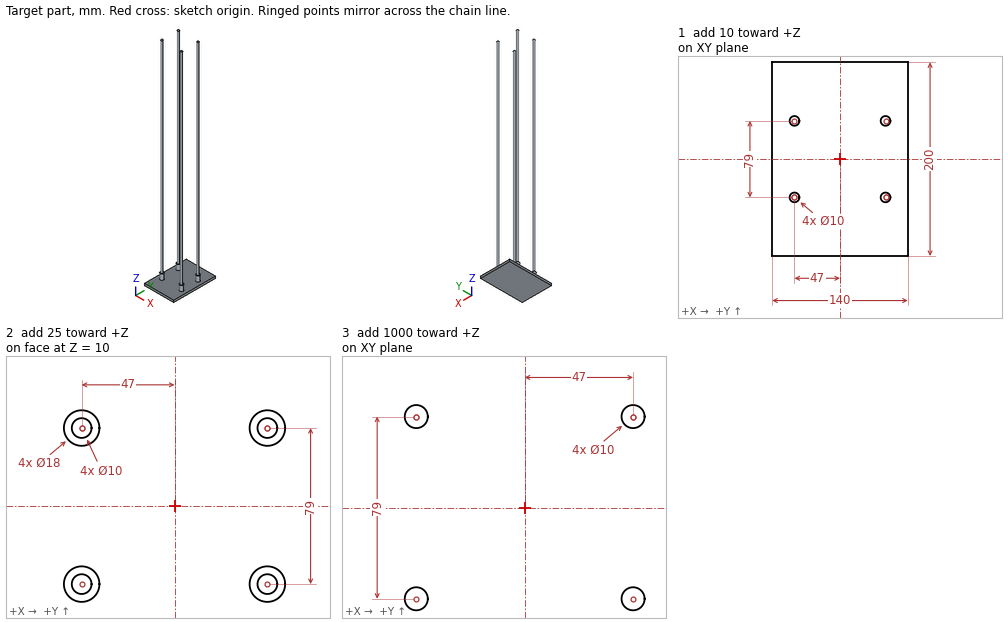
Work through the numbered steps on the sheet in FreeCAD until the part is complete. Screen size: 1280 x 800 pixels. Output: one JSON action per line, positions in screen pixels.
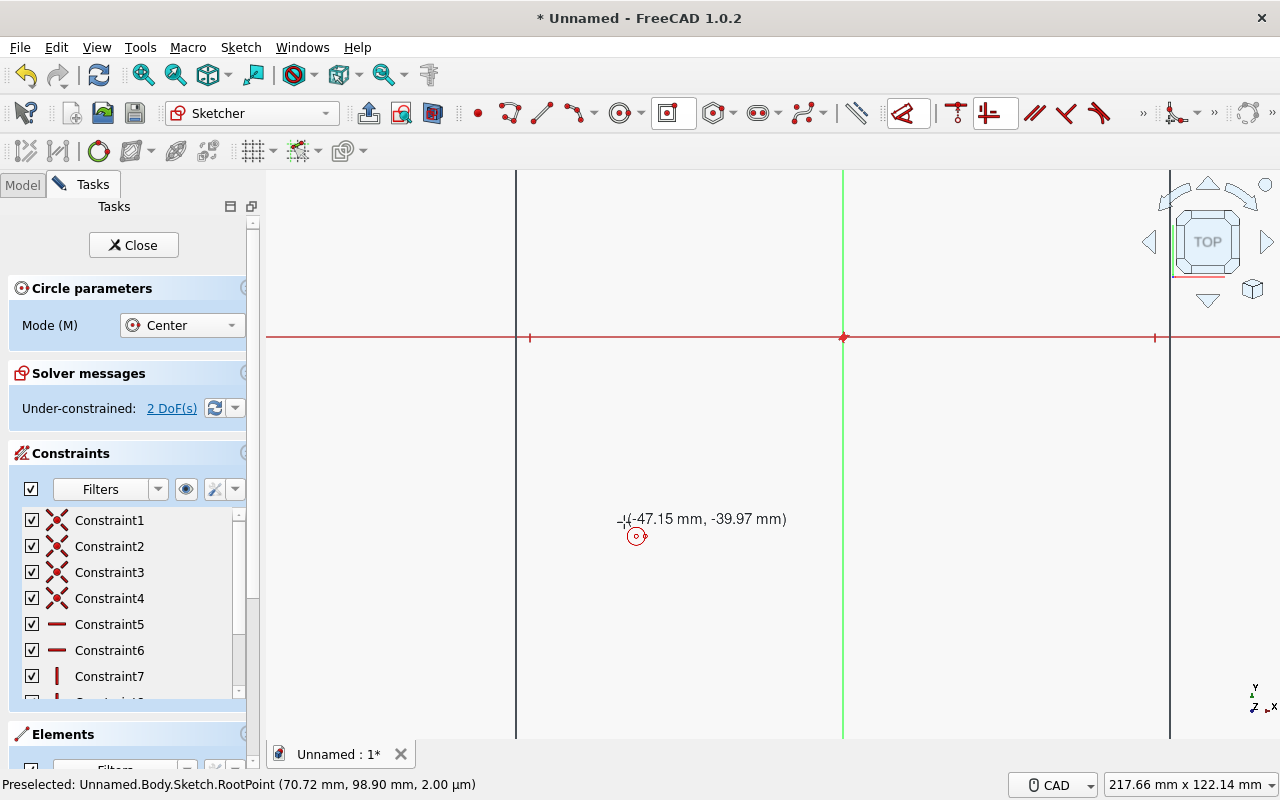
{"action": "left_click", "coordinate": [624, 521]}
{"action": "left_click", "coordinate": [641, 505]}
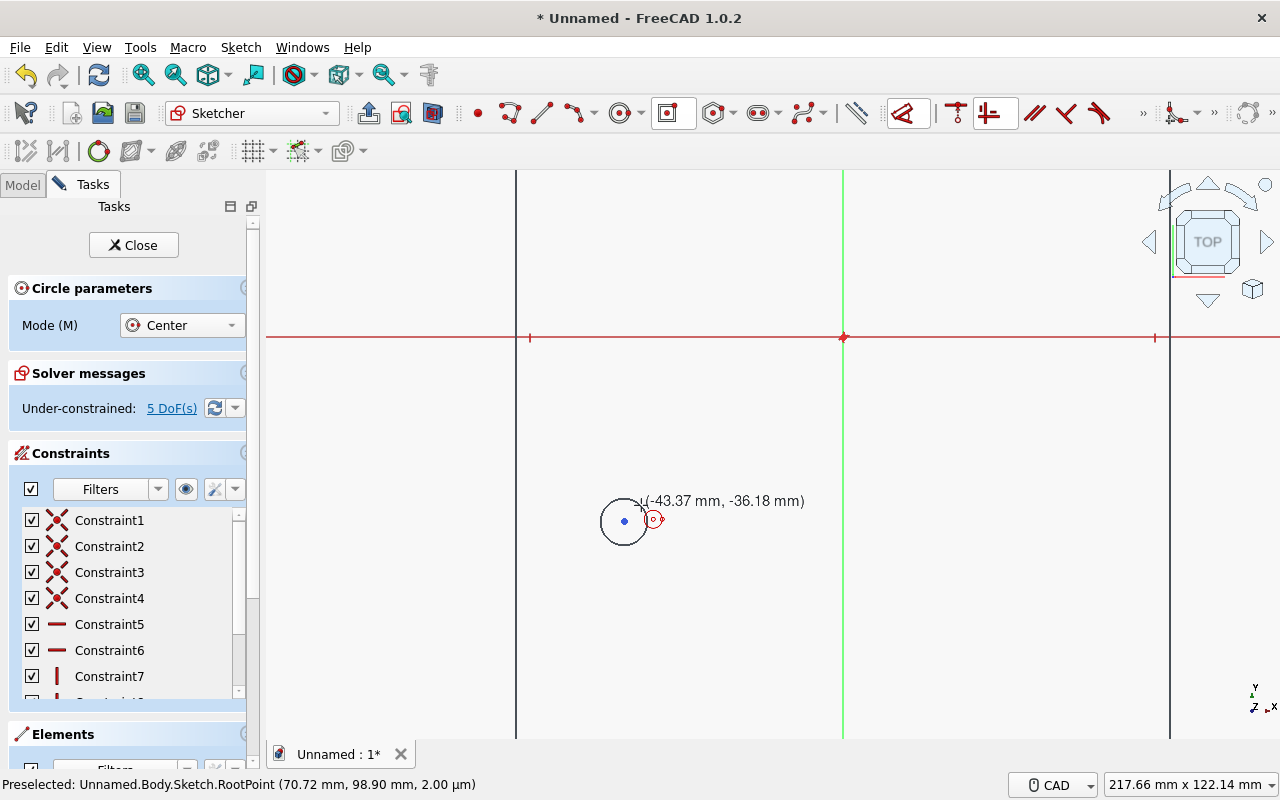
{"action": "left_click", "coordinate": [1062, 521]}
{"action": "left_click", "coordinate": [1078, 505]}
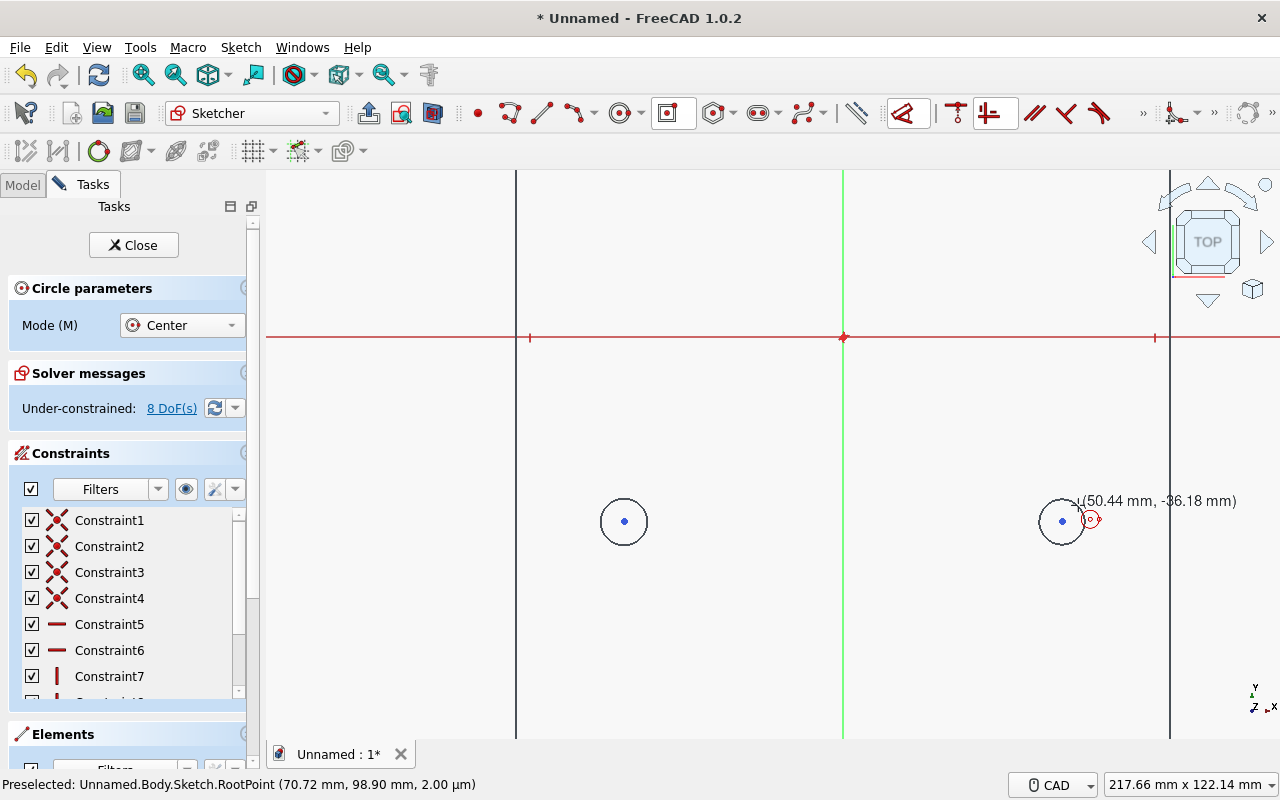
{"action": "scroll", "coordinate": [624, 523], "scroll_direction": "down", "scroll_amount": 5}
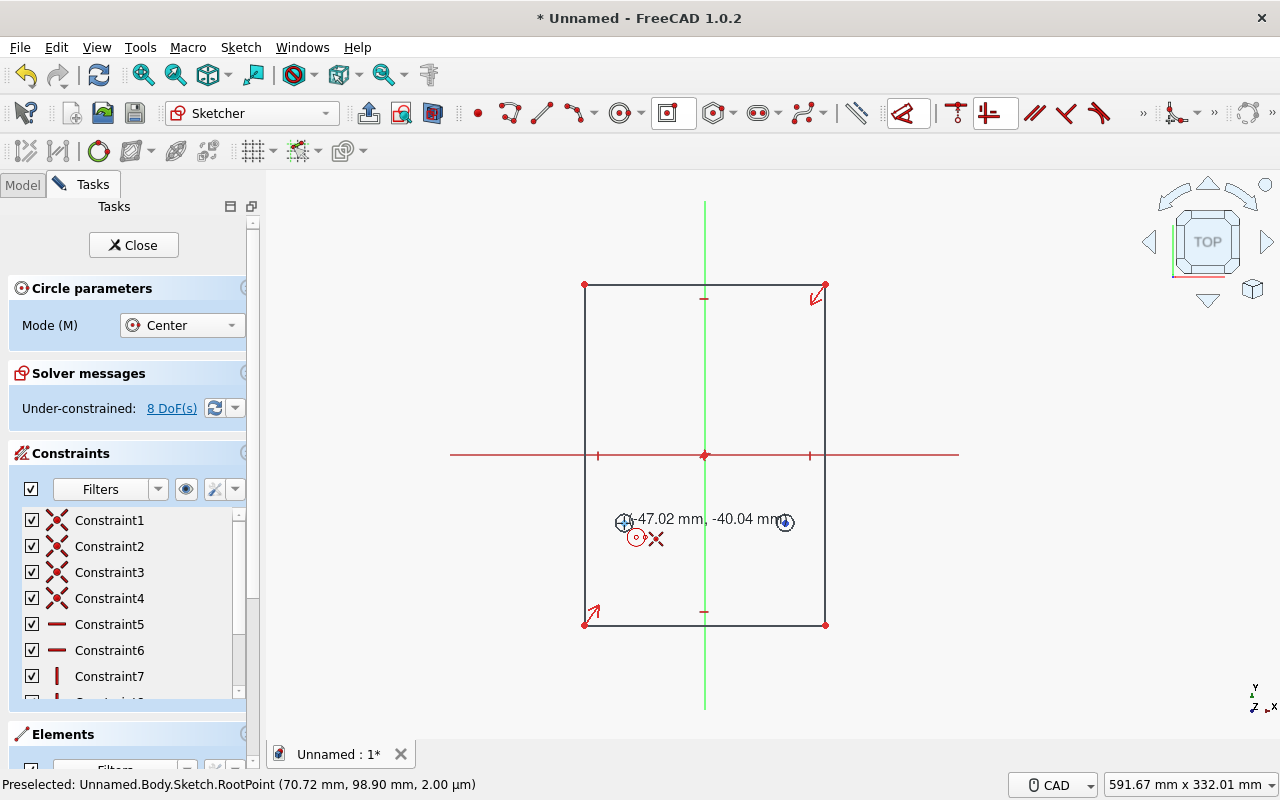
{"action": "scroll", "coordinate": [624, 387], "scroll_direction": "up", "scroll_amount": 5}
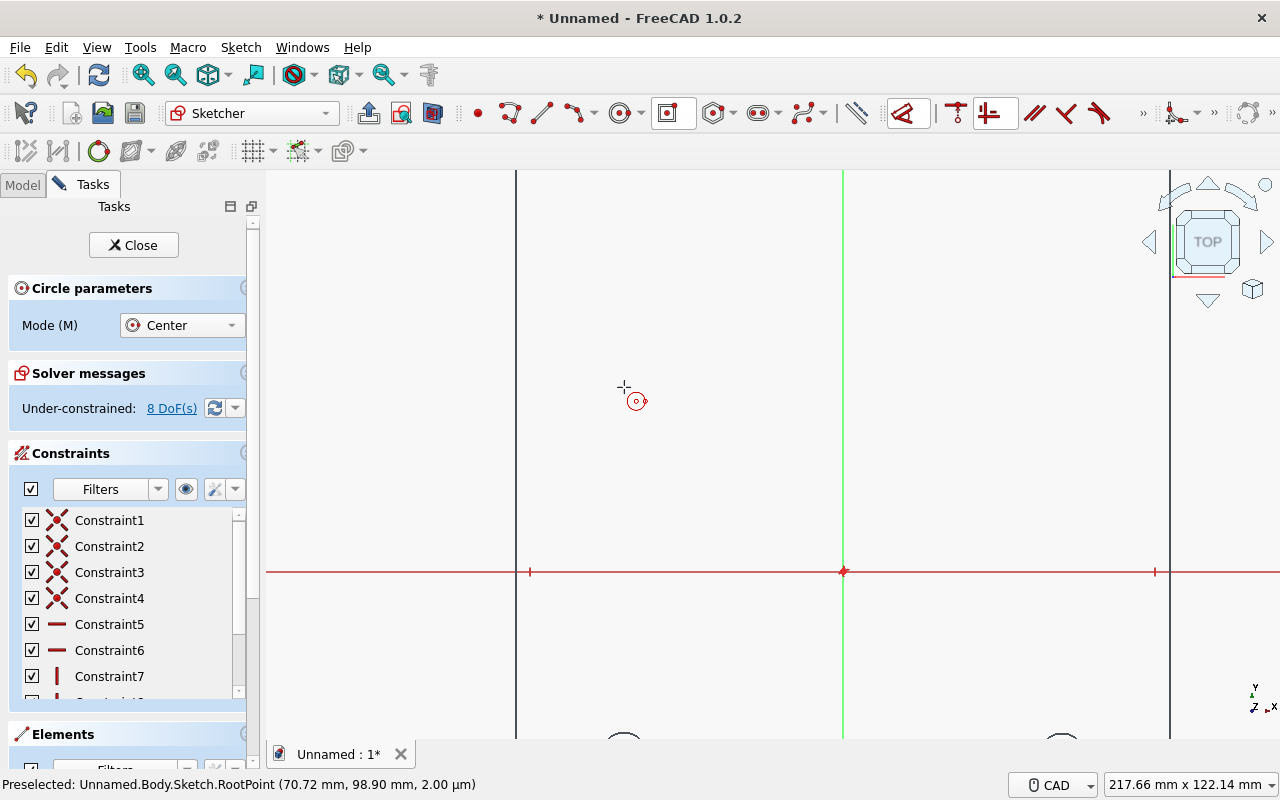
{"action": "left_click", "coordinate": [624, 388]}
{"action": "left_click", "coordinate": [641, 371]}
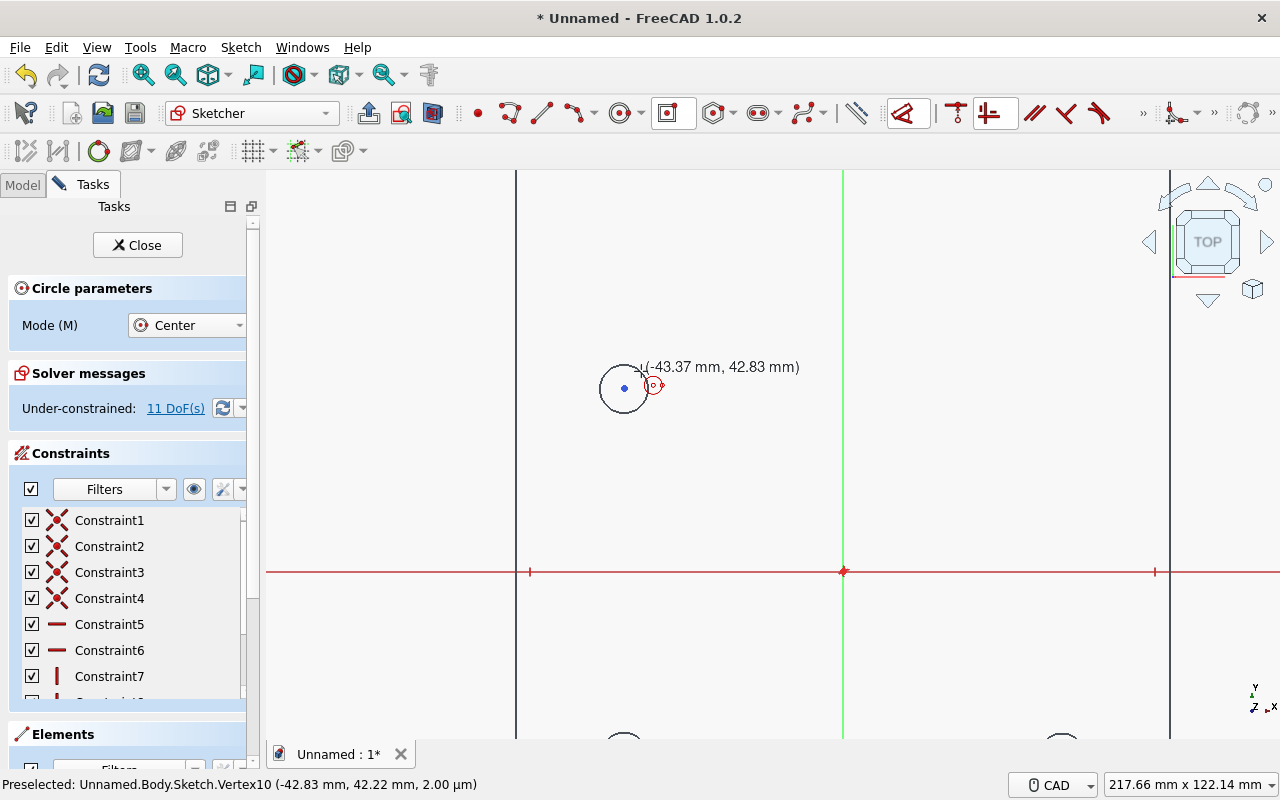
{"action": "left_click", "coordinate": [1062, 388]}
{"action": "left_click", "coordinate": [1078, 371]}
{"action": "key", "text": "Escape"}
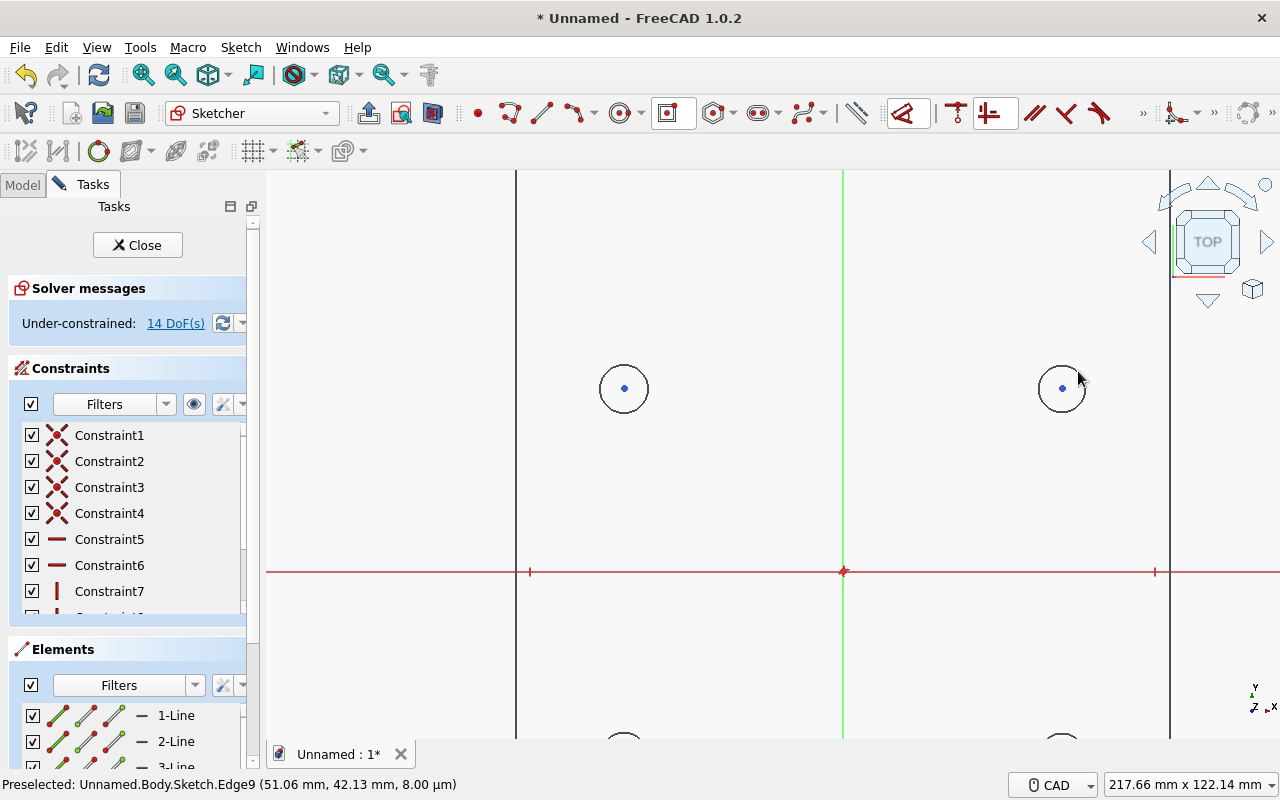
{"action": "scroll", "coordinate": [624, 386], "scroll_direction": "down", "scroll_amount": 5}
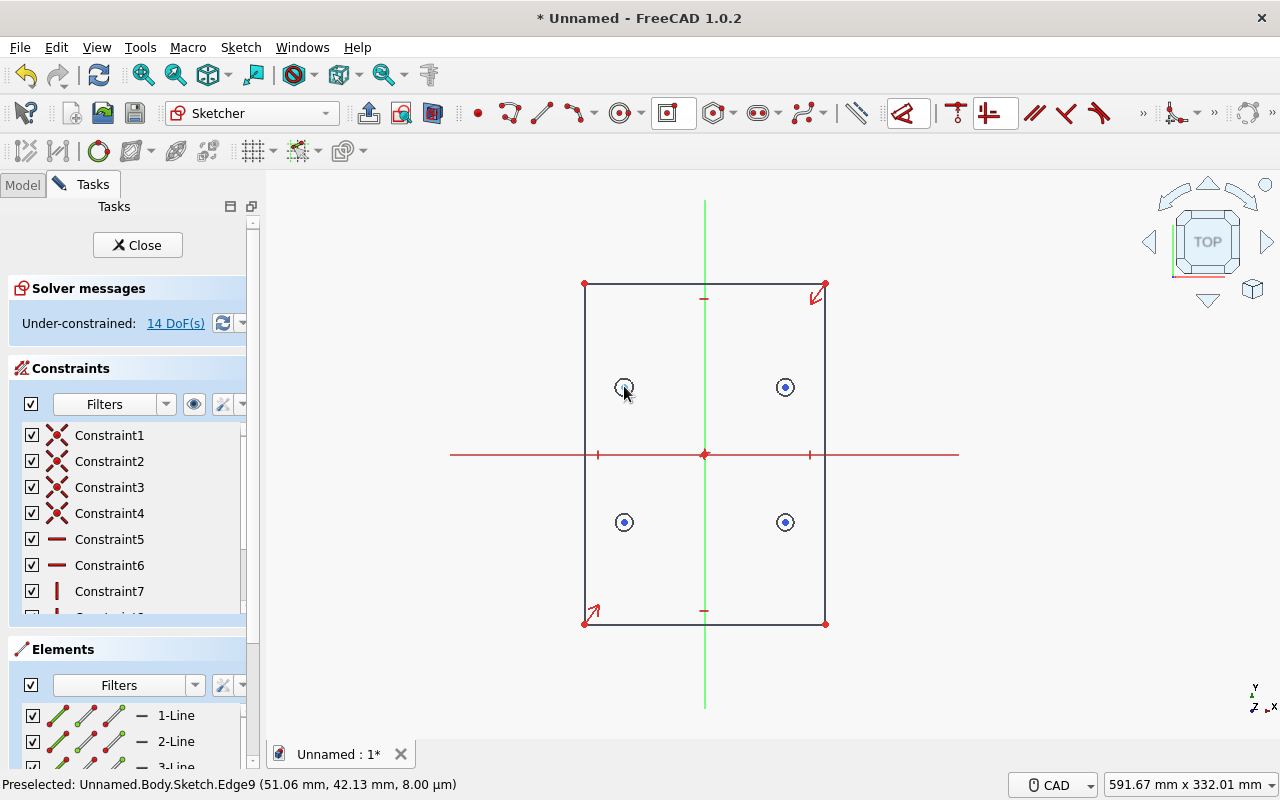
{"action": "scroll", "coordinate": [630, 516], "scroll_direction": "up", "scroll_amount": 3}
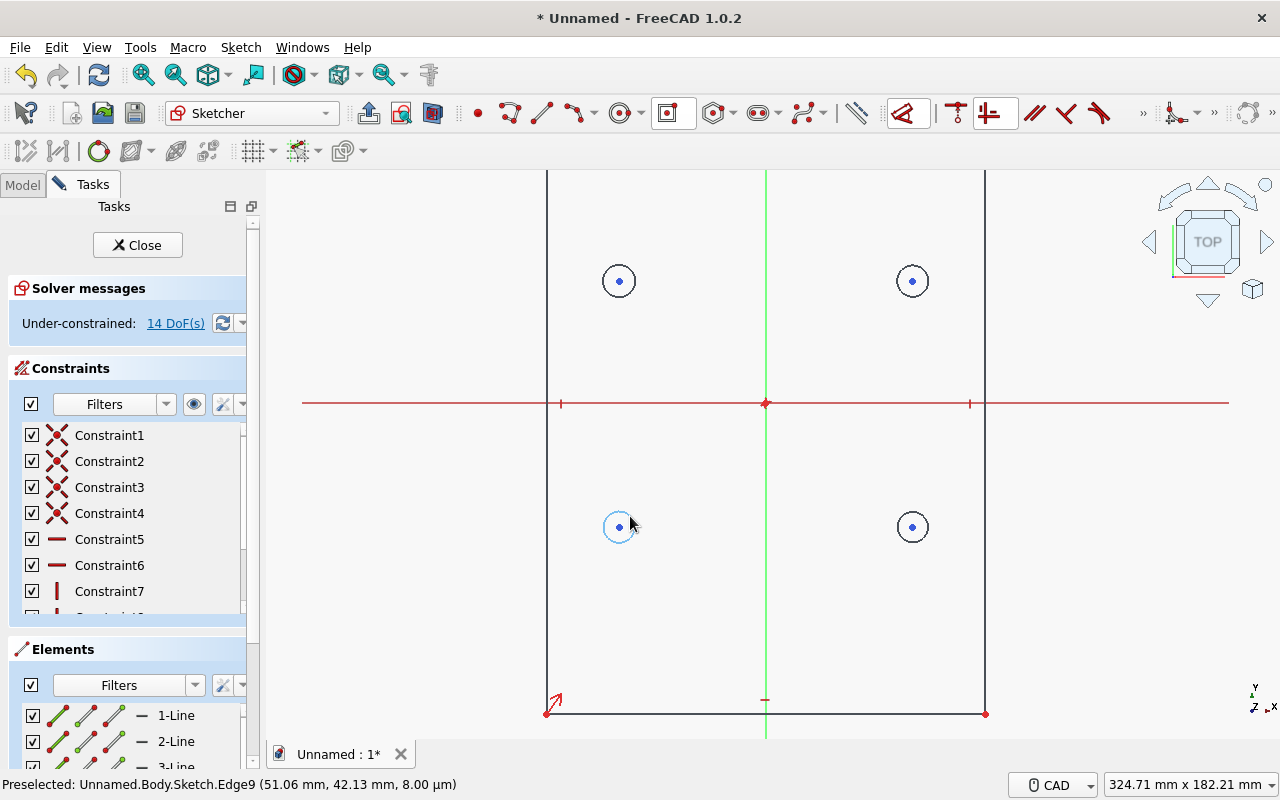
{"action": "left_click", "coordinate": [630, 516]}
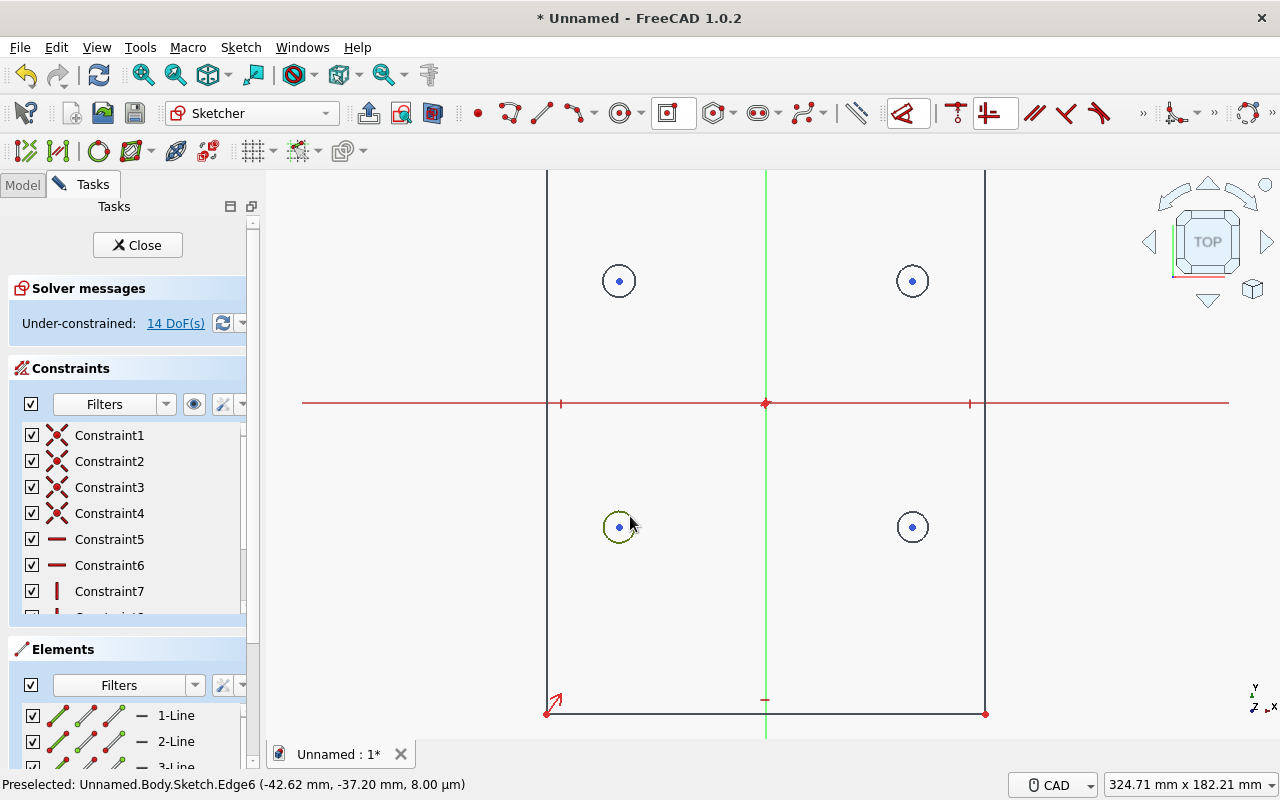
{"action": "left_click", "coordinate": [923, 516]}